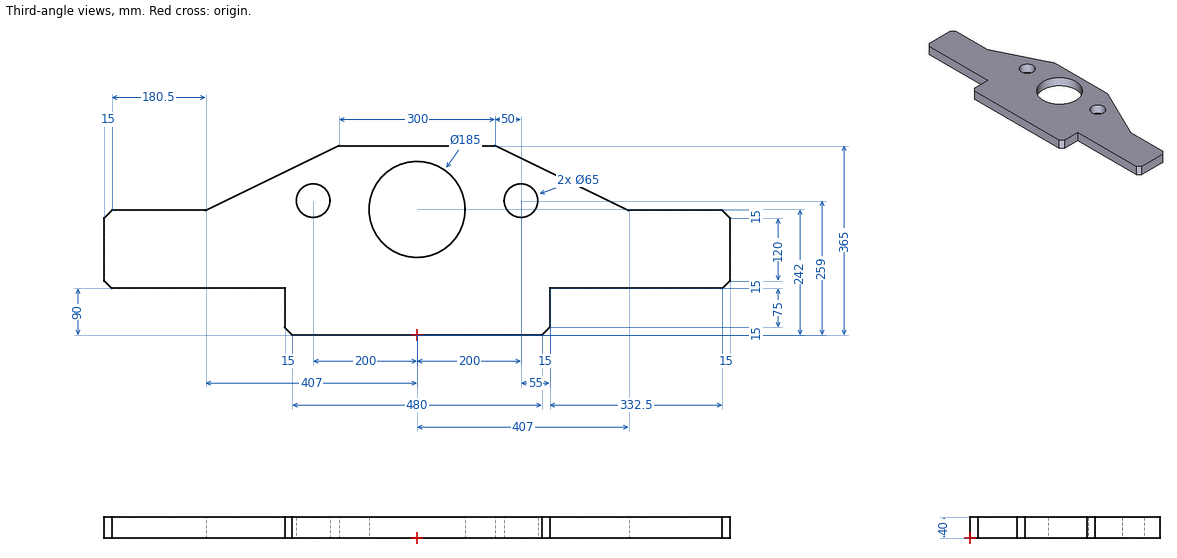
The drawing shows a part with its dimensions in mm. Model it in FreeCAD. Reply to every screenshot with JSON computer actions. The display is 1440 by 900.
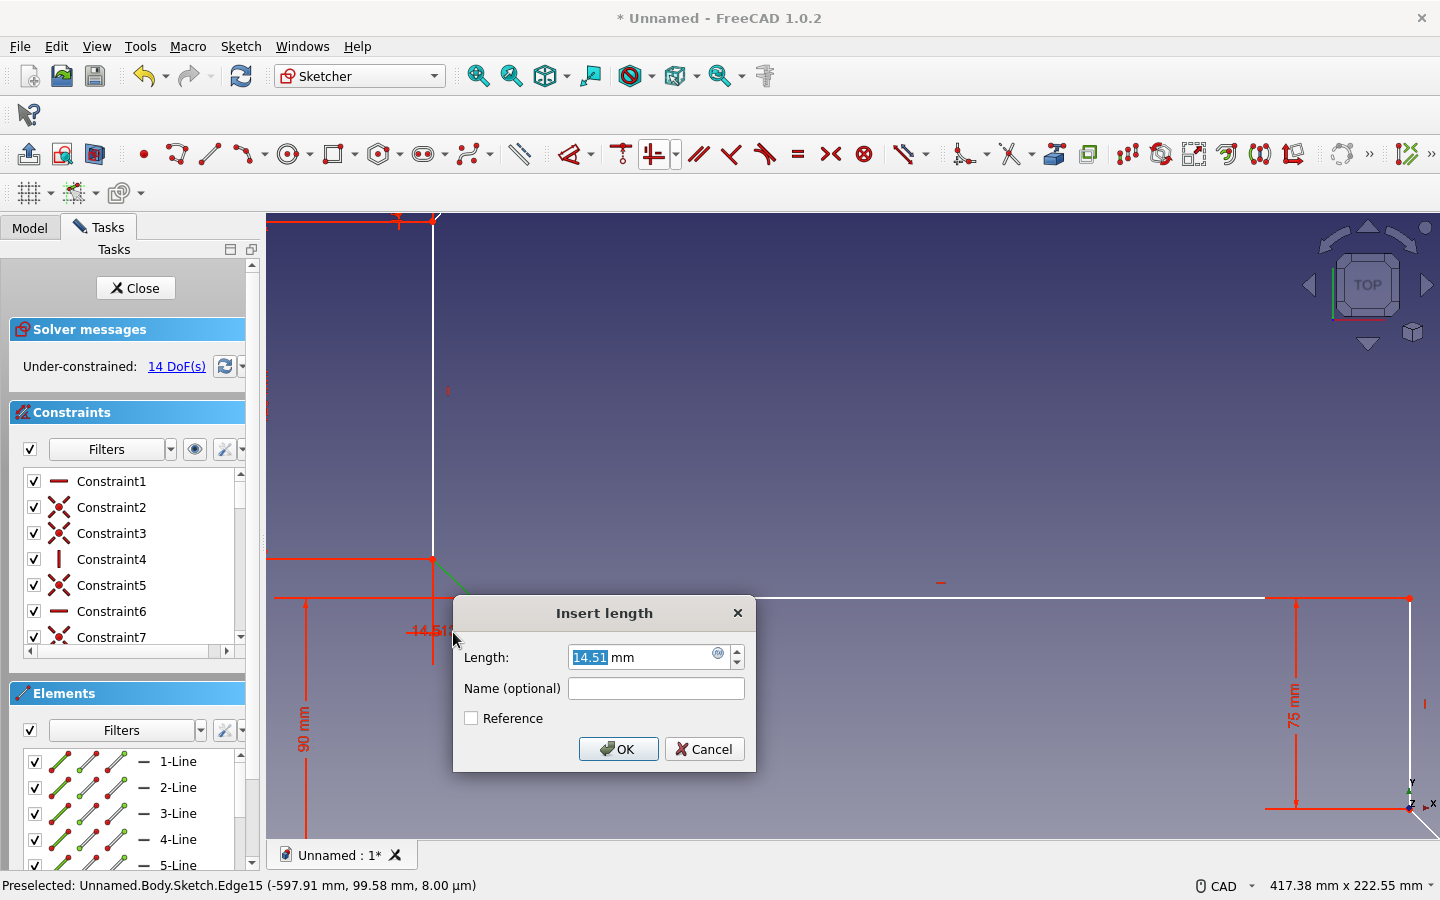
{"action": "type", "text": "15"}
{"action": "key", "text": "Return"}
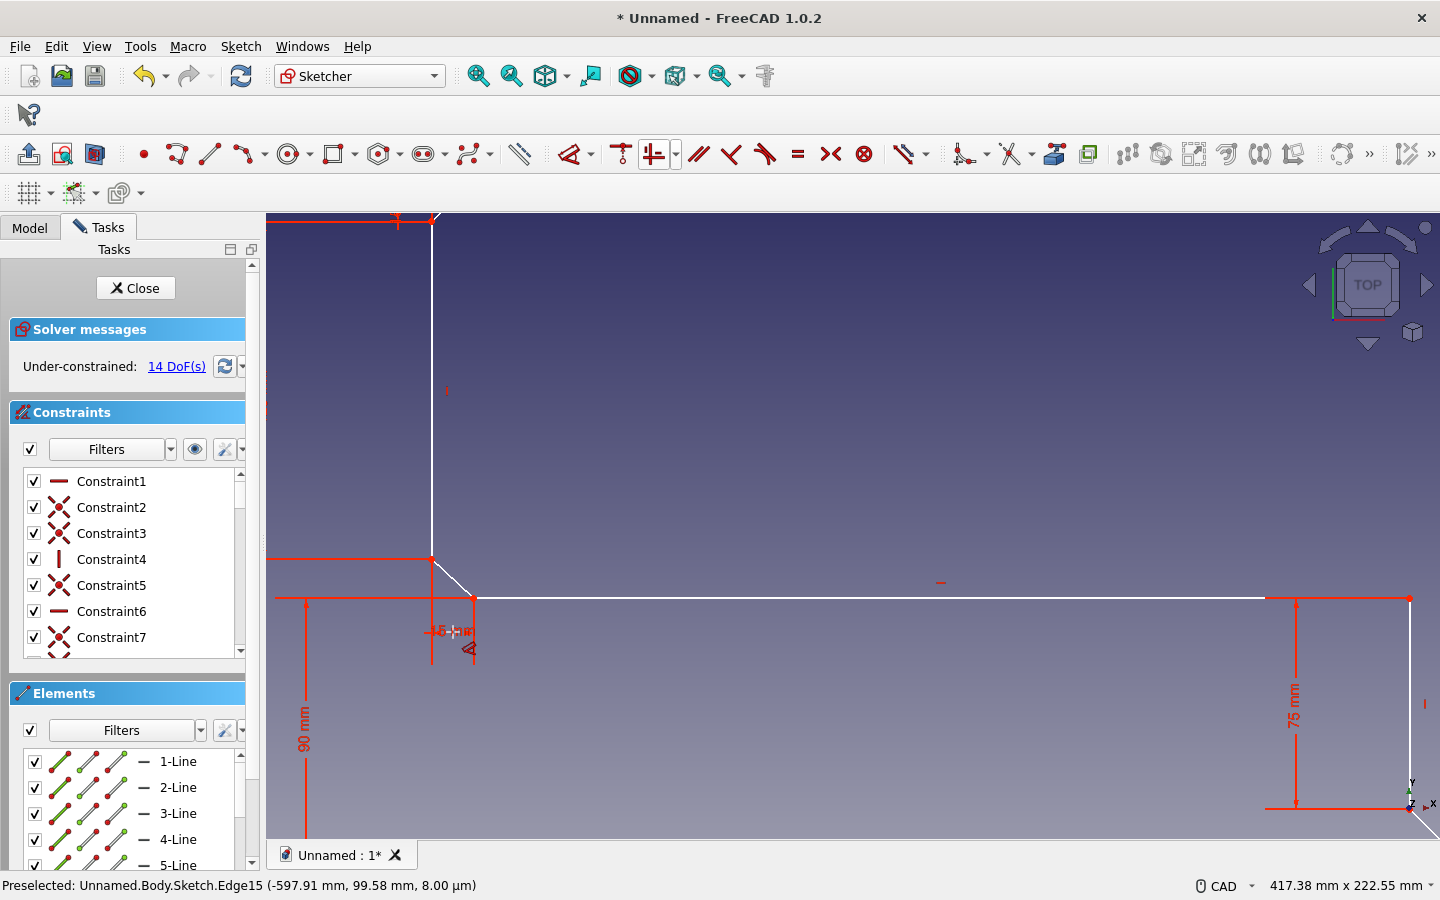
{"action": "left_click", "coordinate": [444, 571]}
{"action": "left_click", "coordinate": [398, 579]}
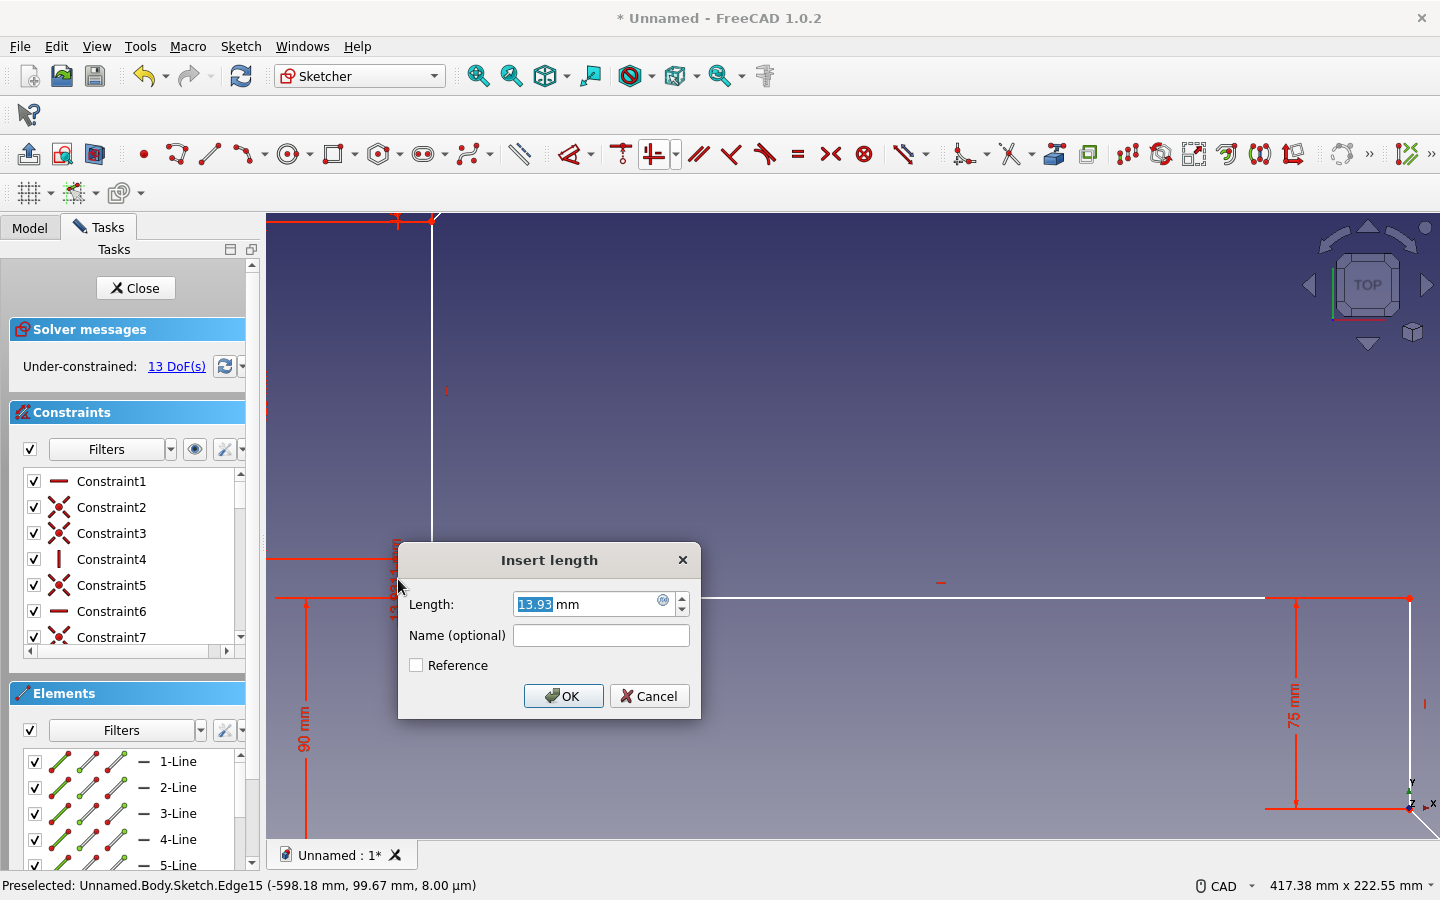
{"action": "type", "text": "15"}
{"action": "key", "text": "Return"}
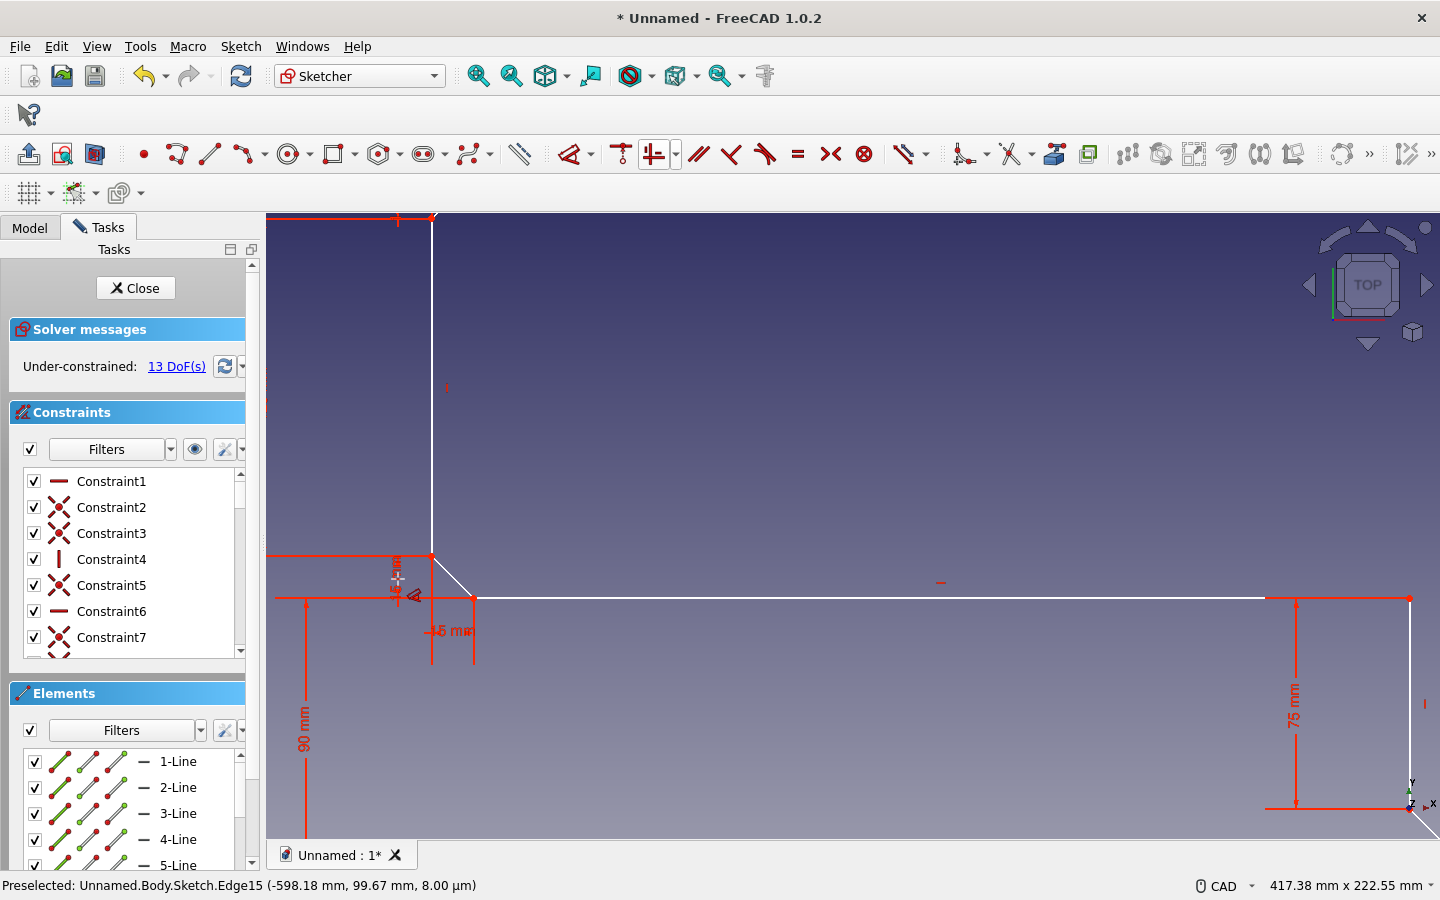
{"action": "scroll", "coordinate": [445, 573], "scroll_direction": "down", "scroll_amount": 8}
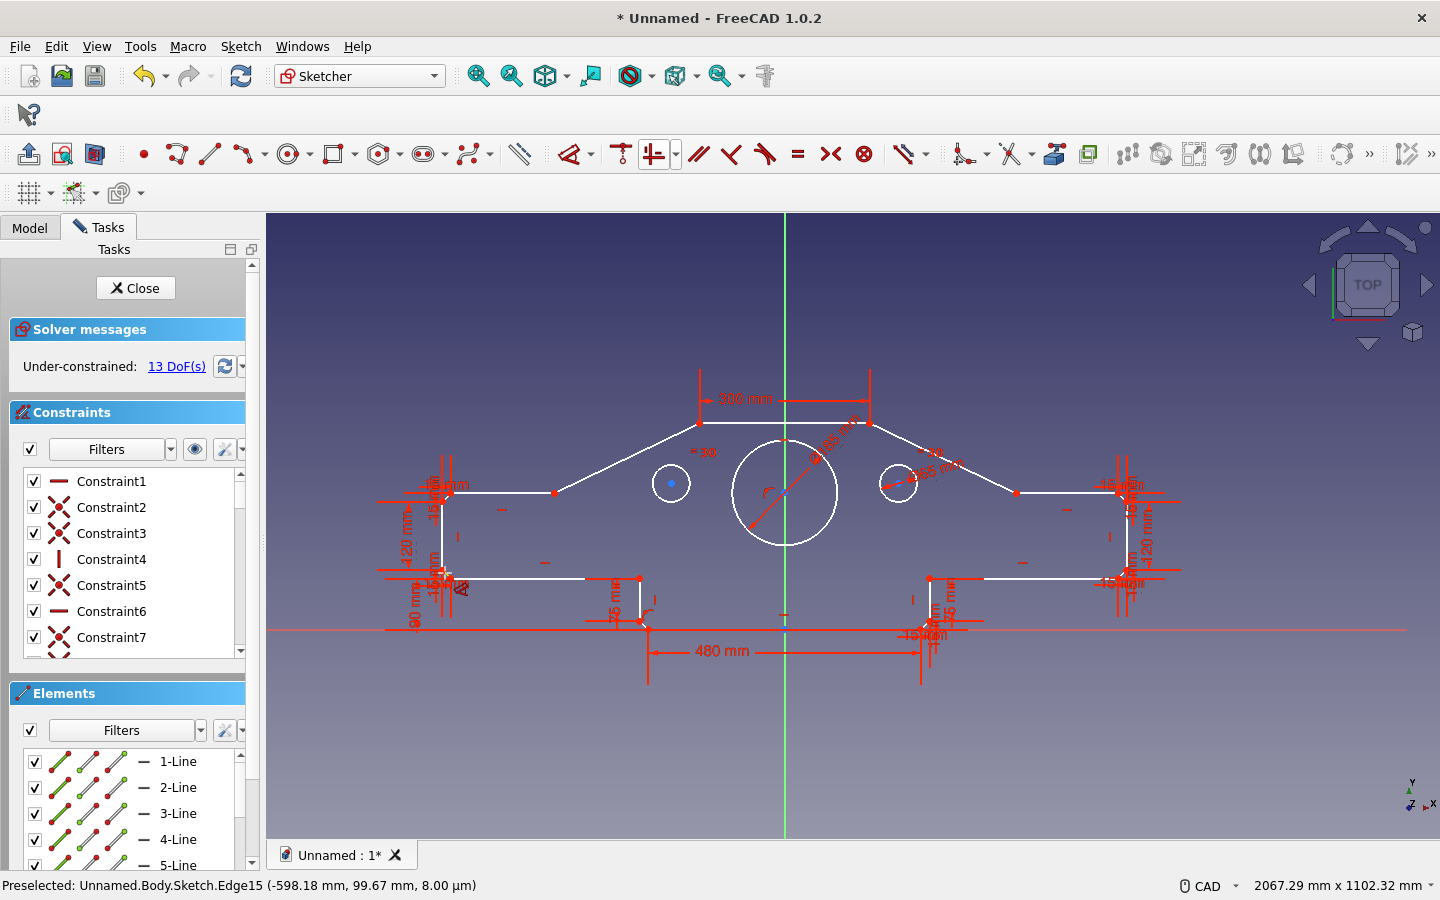
{"action": "scroll", "coordinate": [642, 624], "scroll_direction": "up", "scroll_amount": 8}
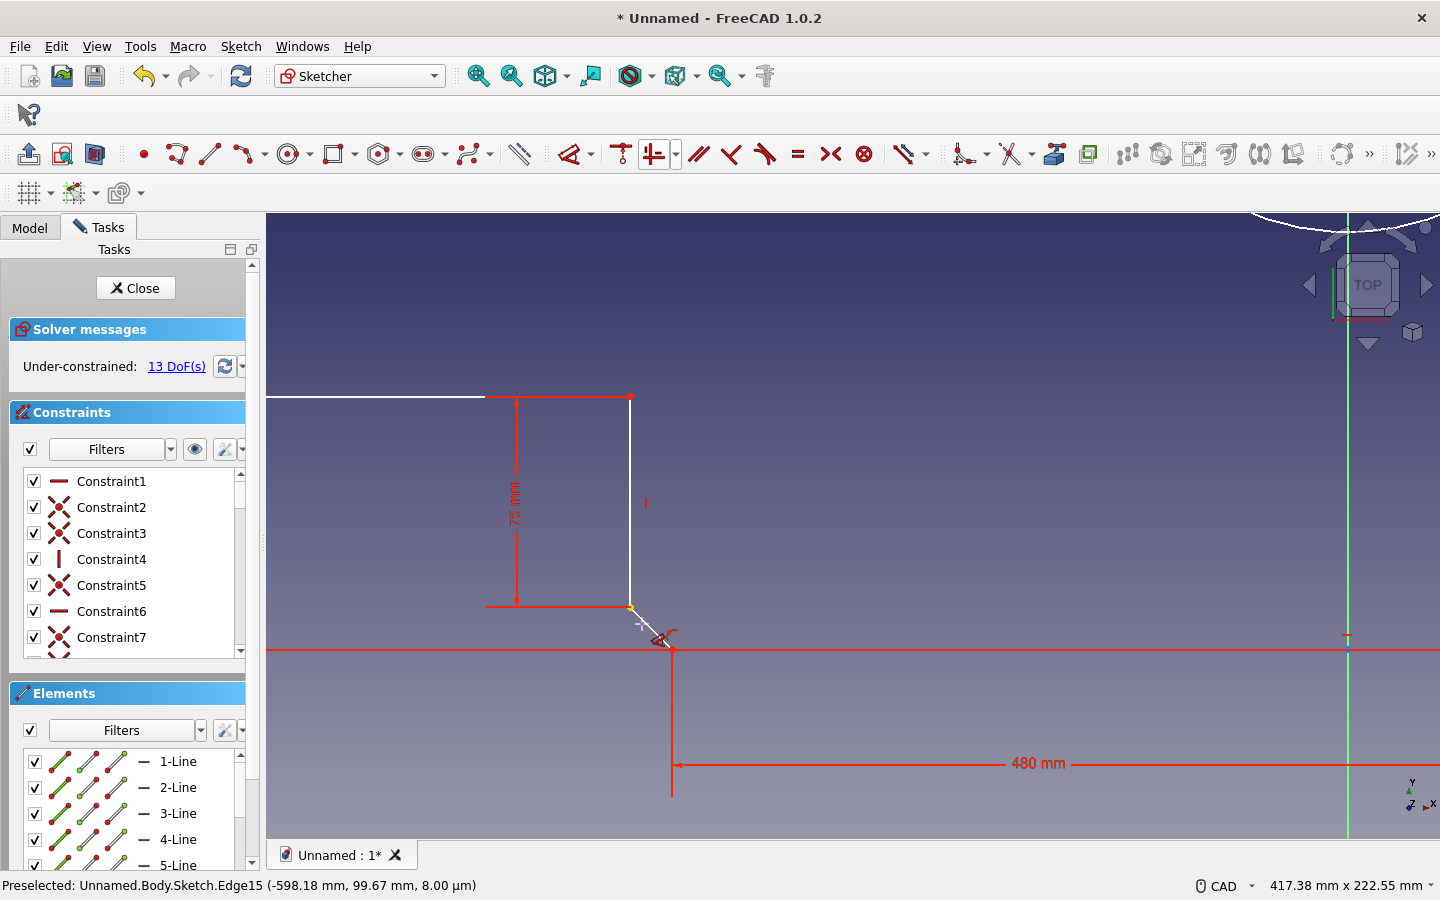
{"action": "left_click", "coordinate": [643, 620]}
{"action": "left_click", "coordinate": [651, 684]}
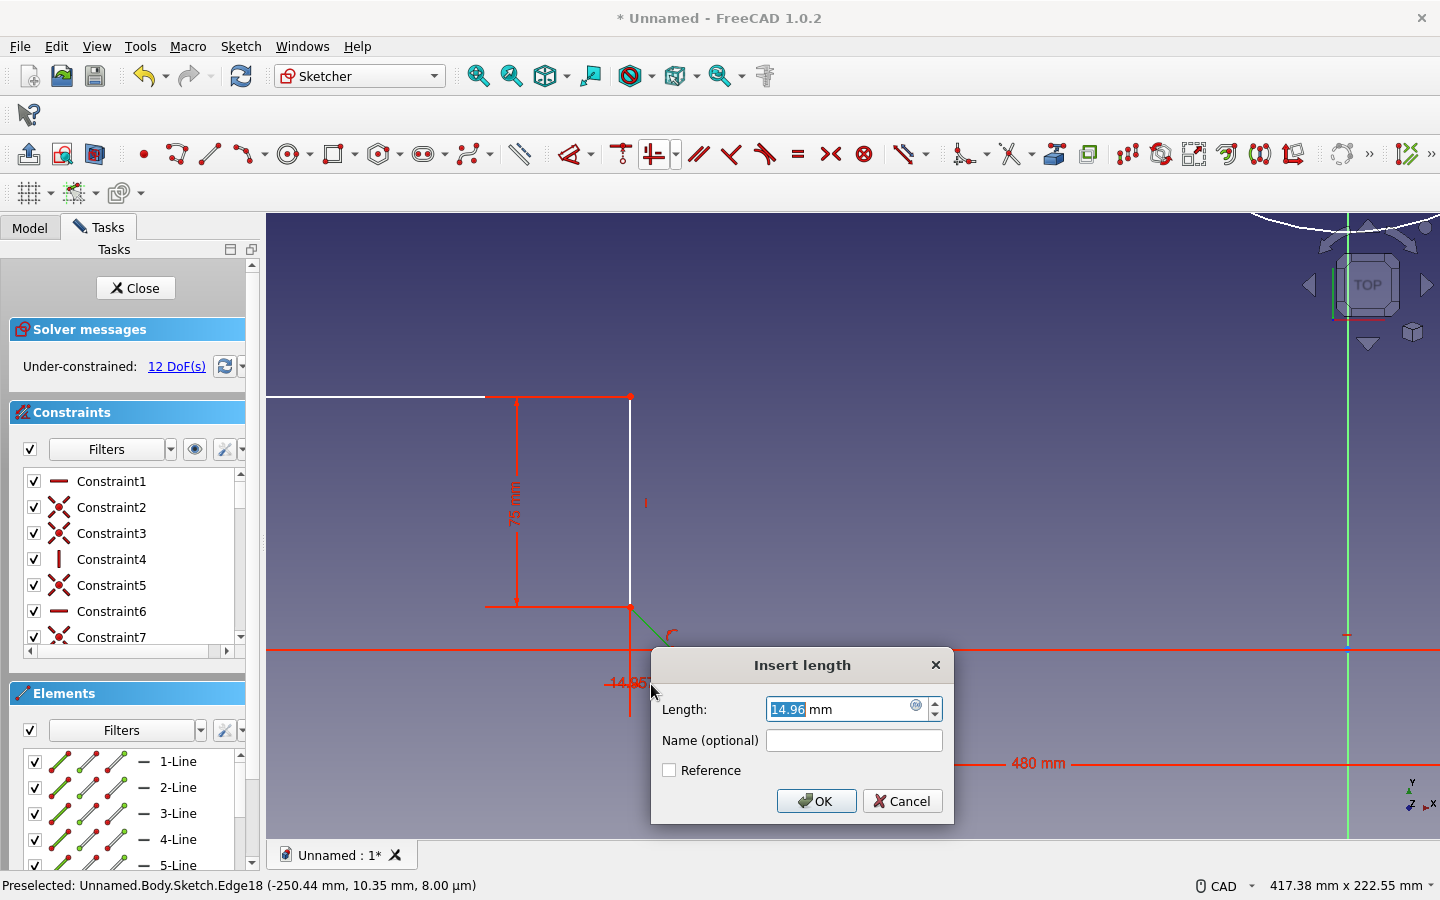
{"action": "type", "text": "15"}
{"action": "key", "text": "Return"}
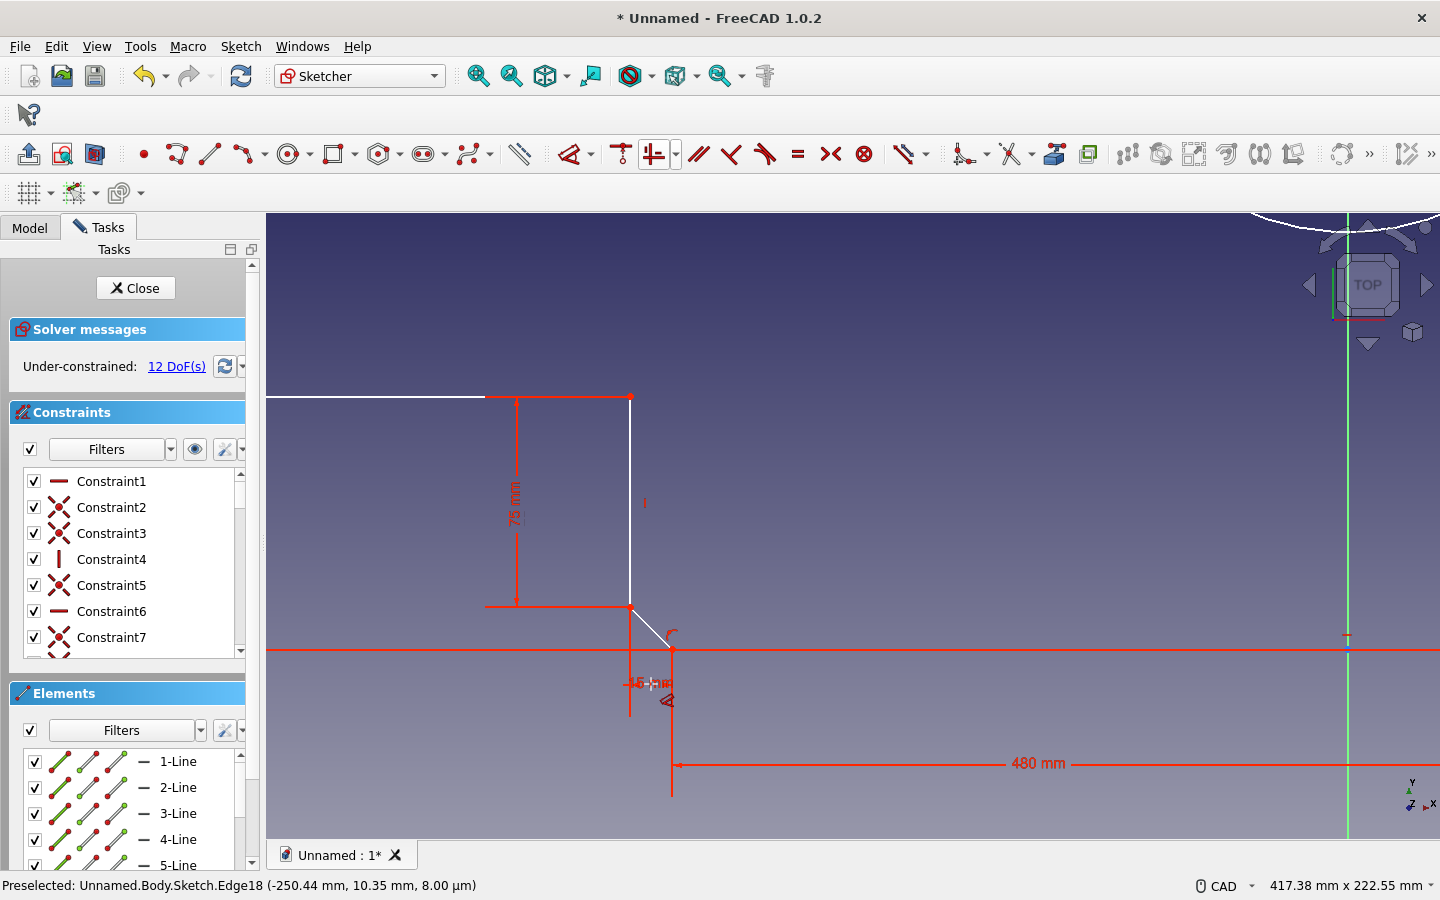
{"action": "scroll", "coordinate": [642, 625], "scroll_direction": "down", "scroll_amount": 8}